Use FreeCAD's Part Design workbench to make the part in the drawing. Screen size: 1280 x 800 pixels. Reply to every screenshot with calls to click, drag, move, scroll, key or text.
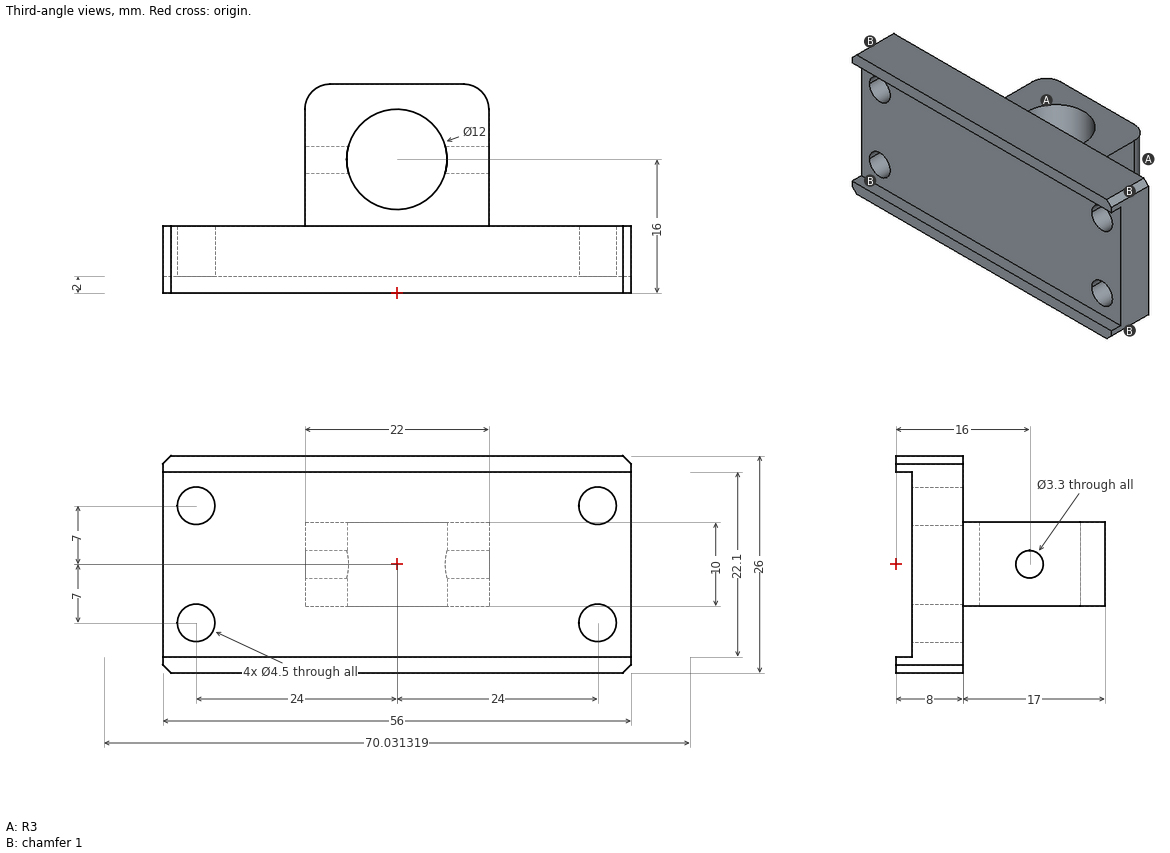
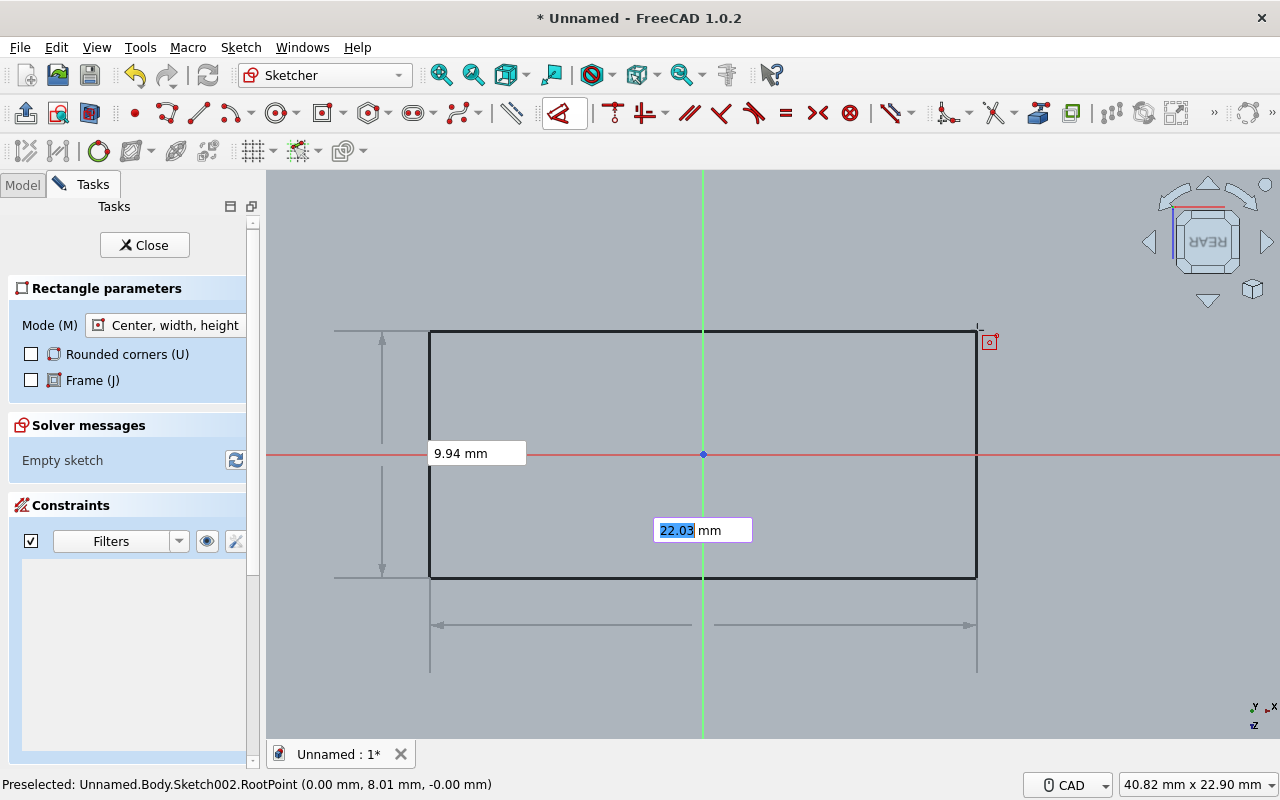
text(22)
key(Tab)
text(10)
key(Return)
key(Escape)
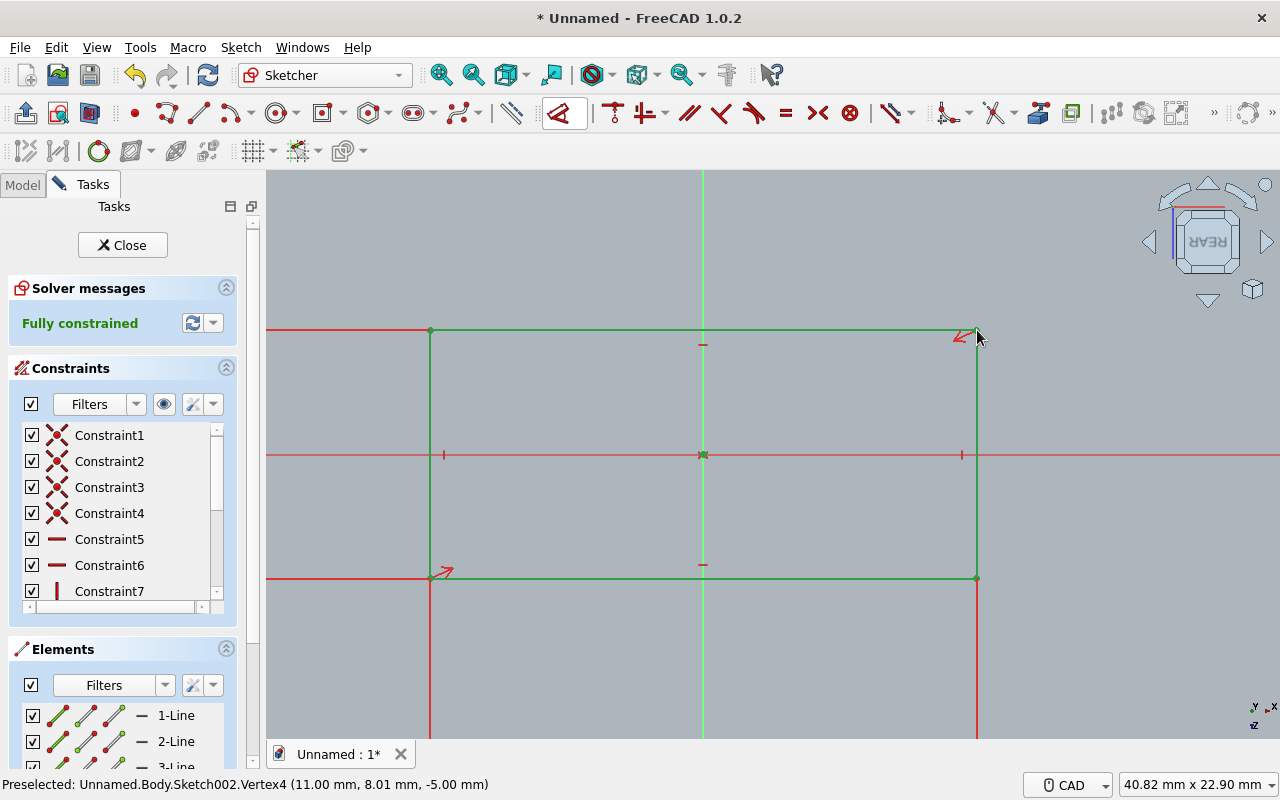
click(123, 245)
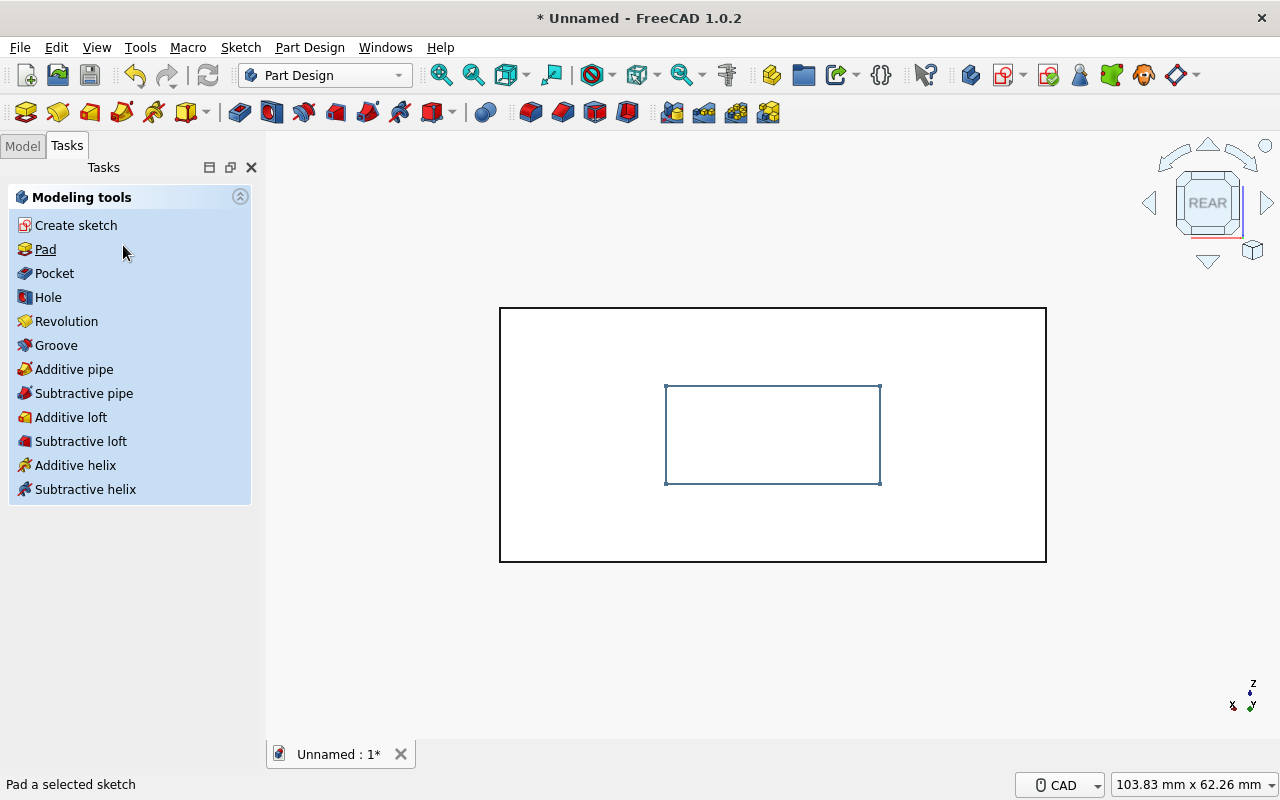
click(26, 112)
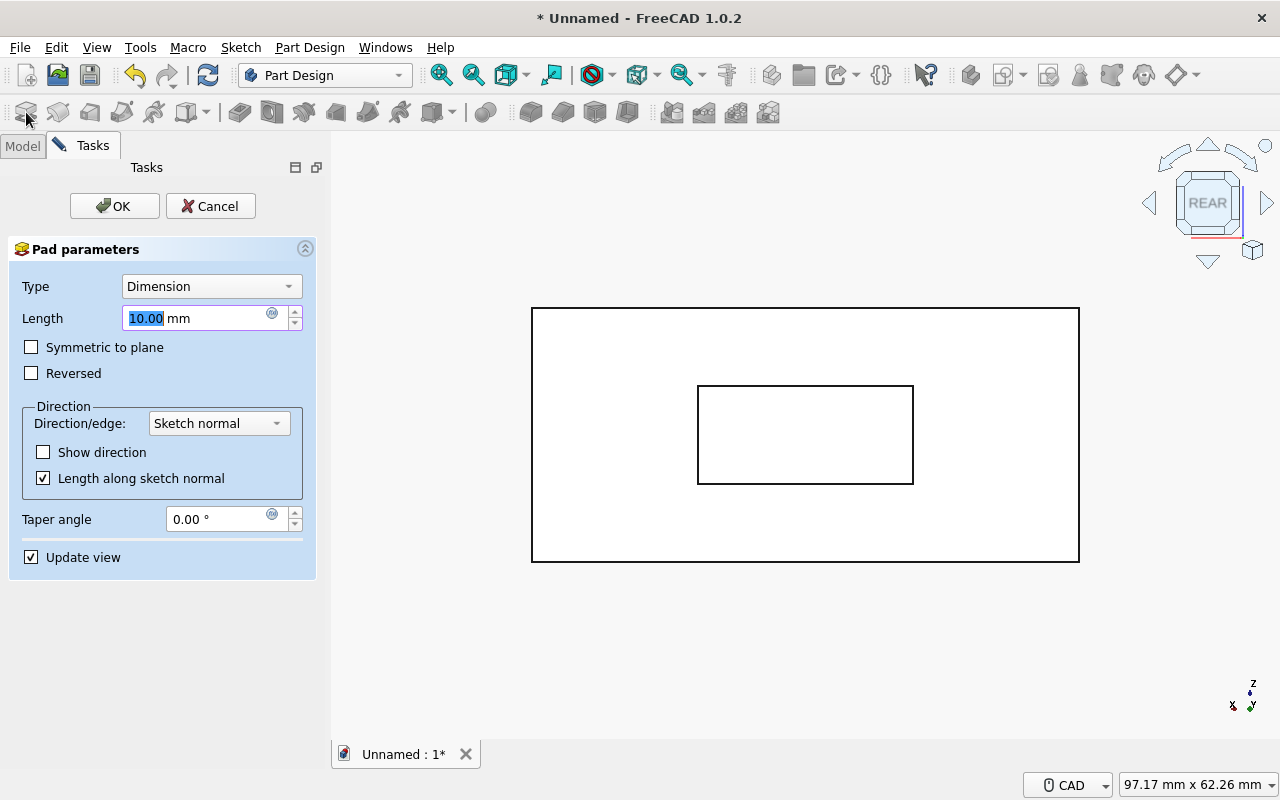
text(17)
key(Tab)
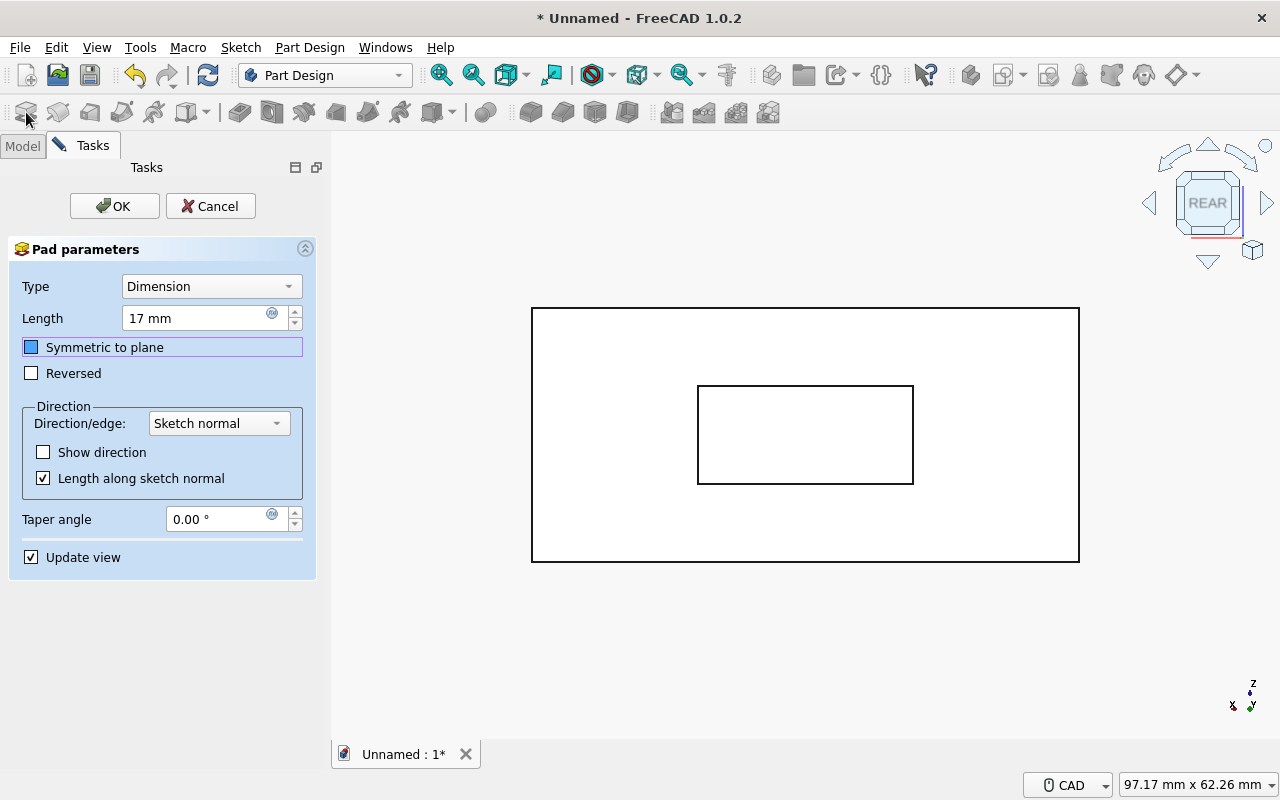
click(115, 206)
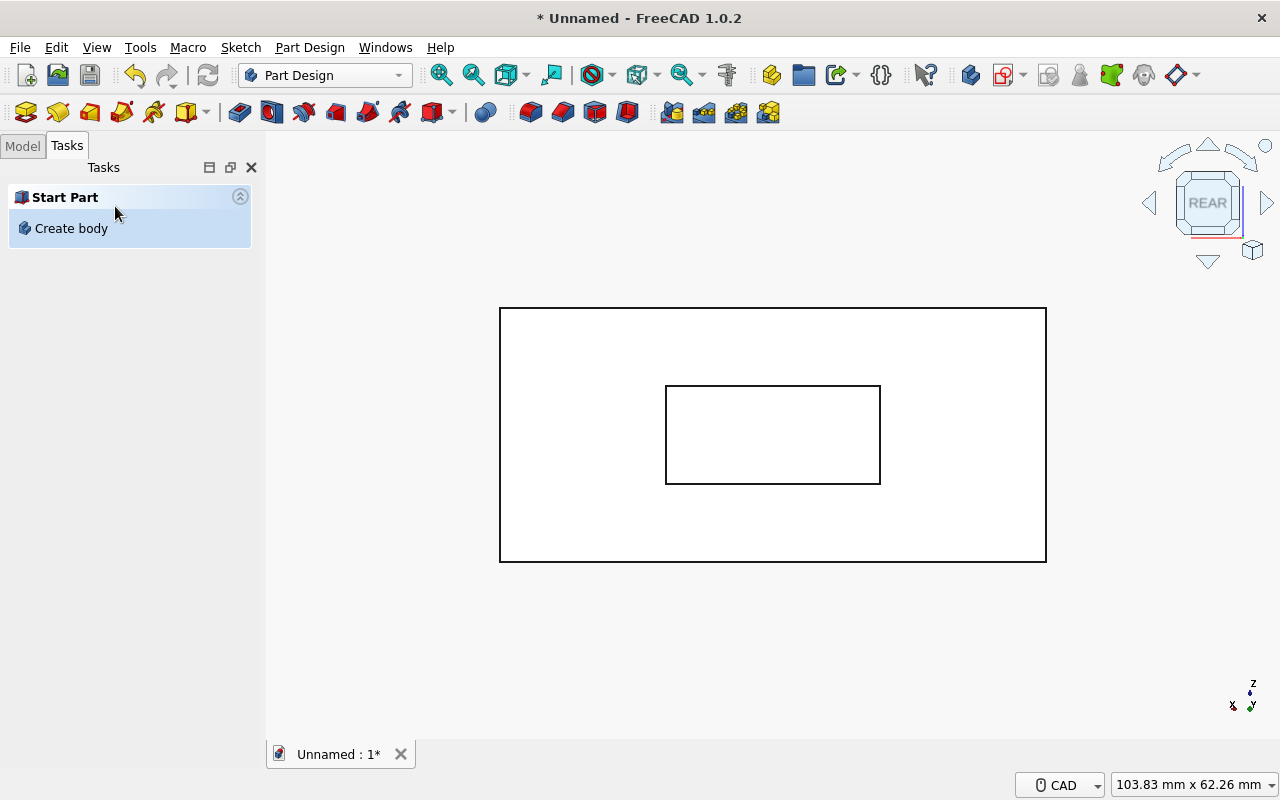
key(5)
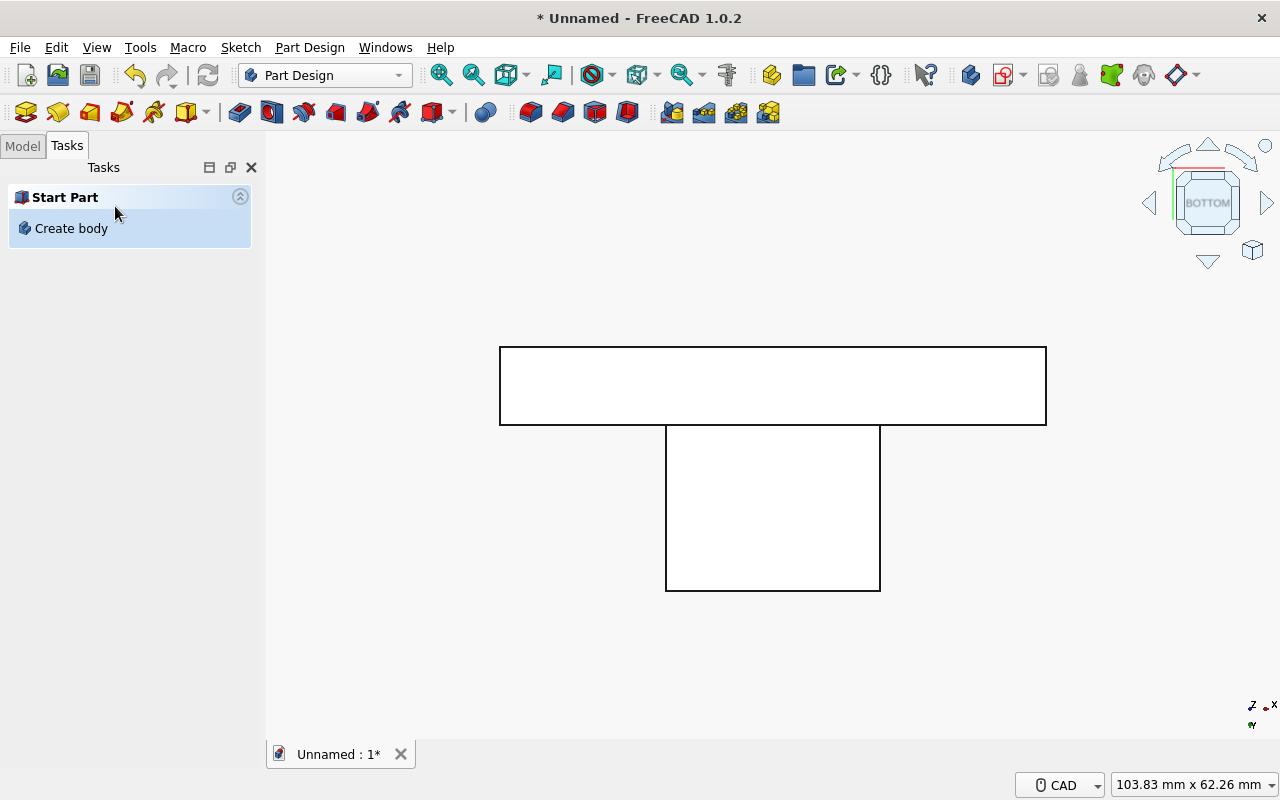
click(1007, 385)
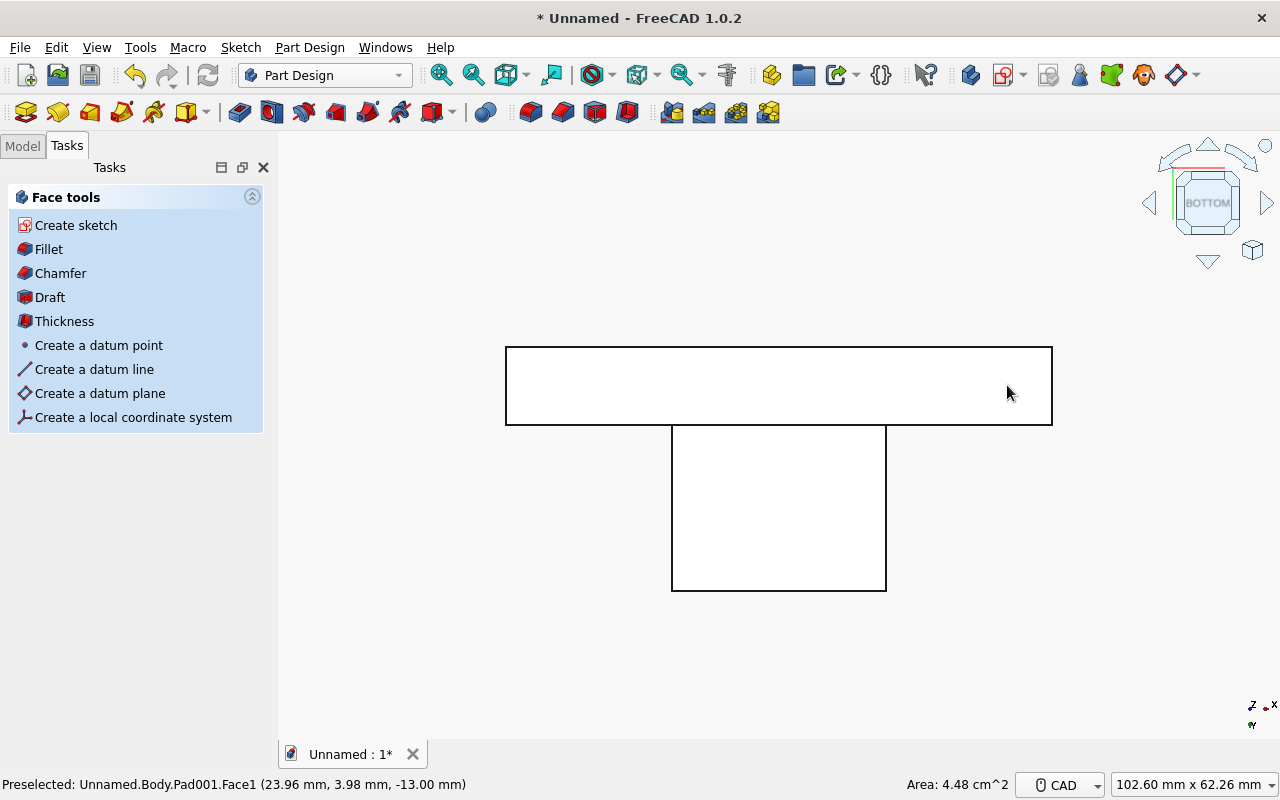
click(1004, 76)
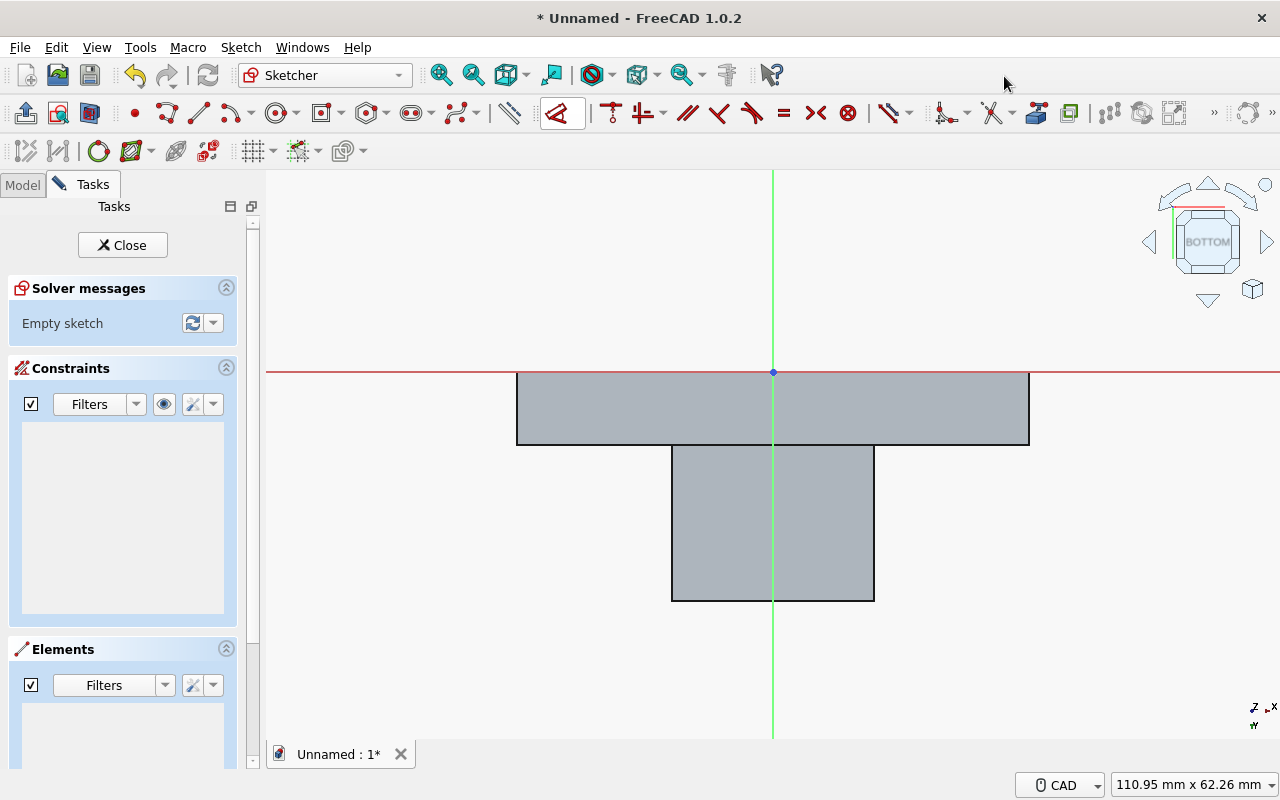
scroll(856, 495, up, 3)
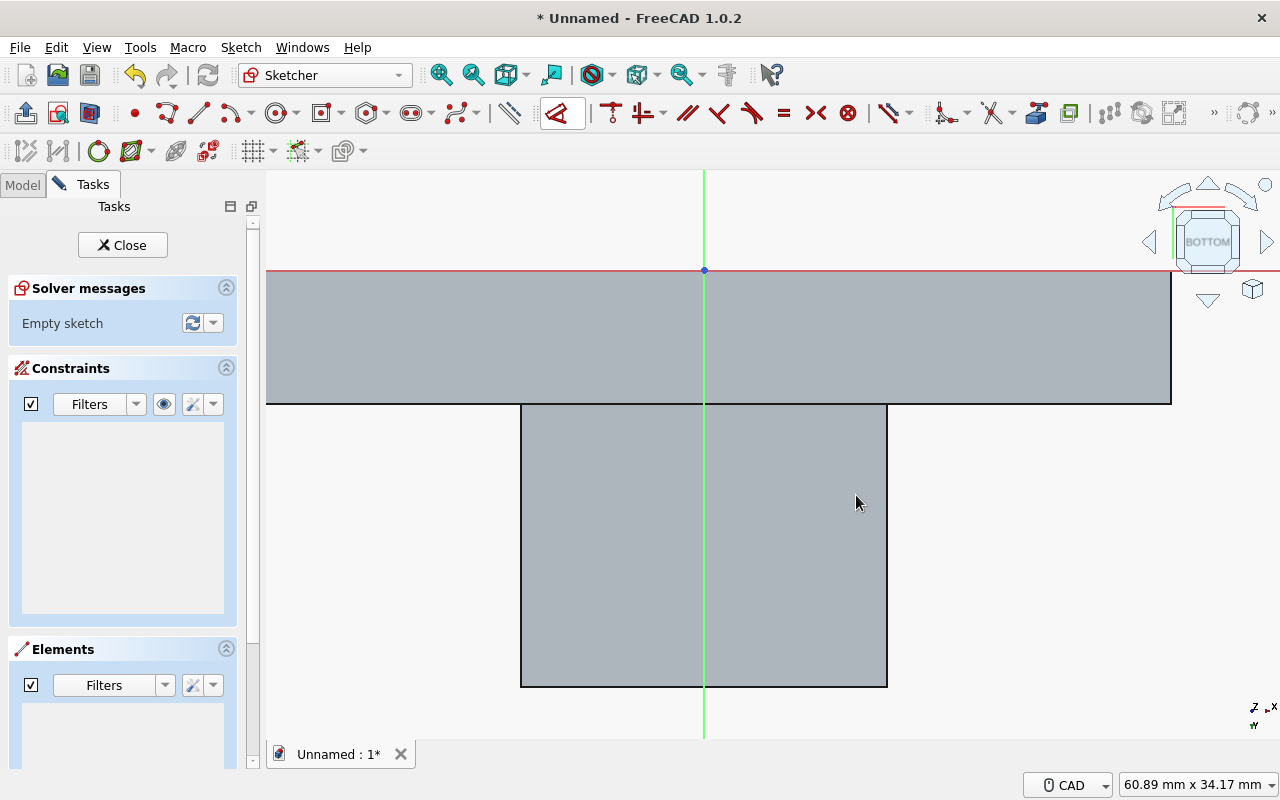
click(276, 114)